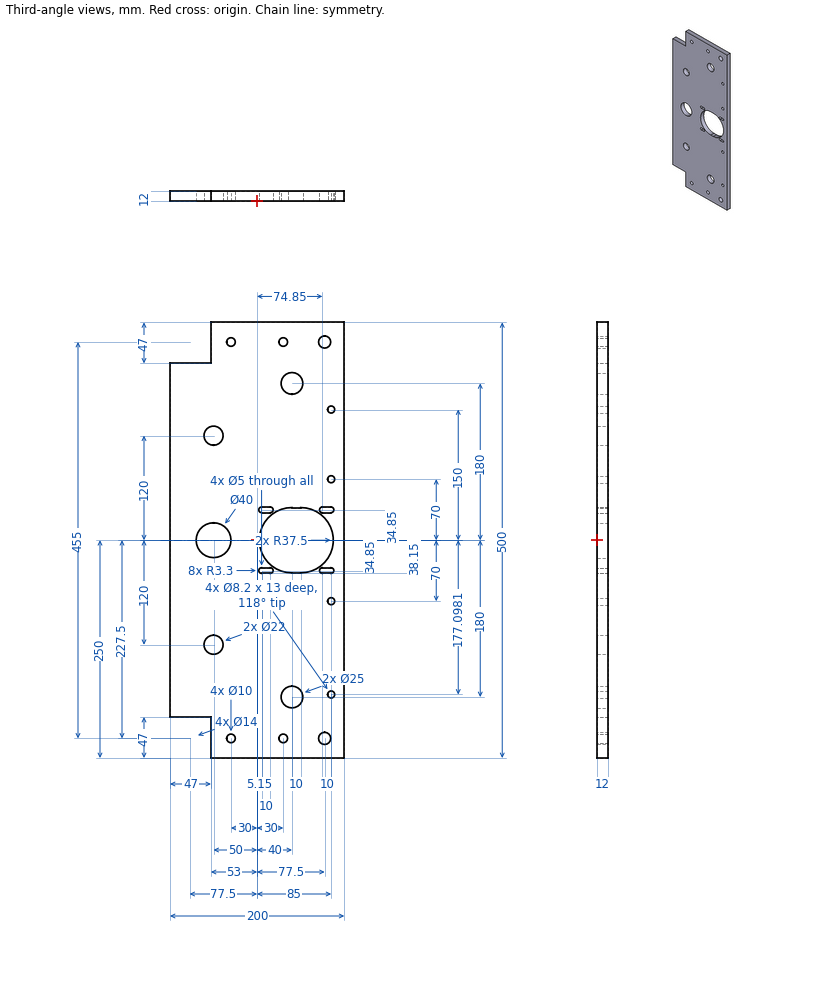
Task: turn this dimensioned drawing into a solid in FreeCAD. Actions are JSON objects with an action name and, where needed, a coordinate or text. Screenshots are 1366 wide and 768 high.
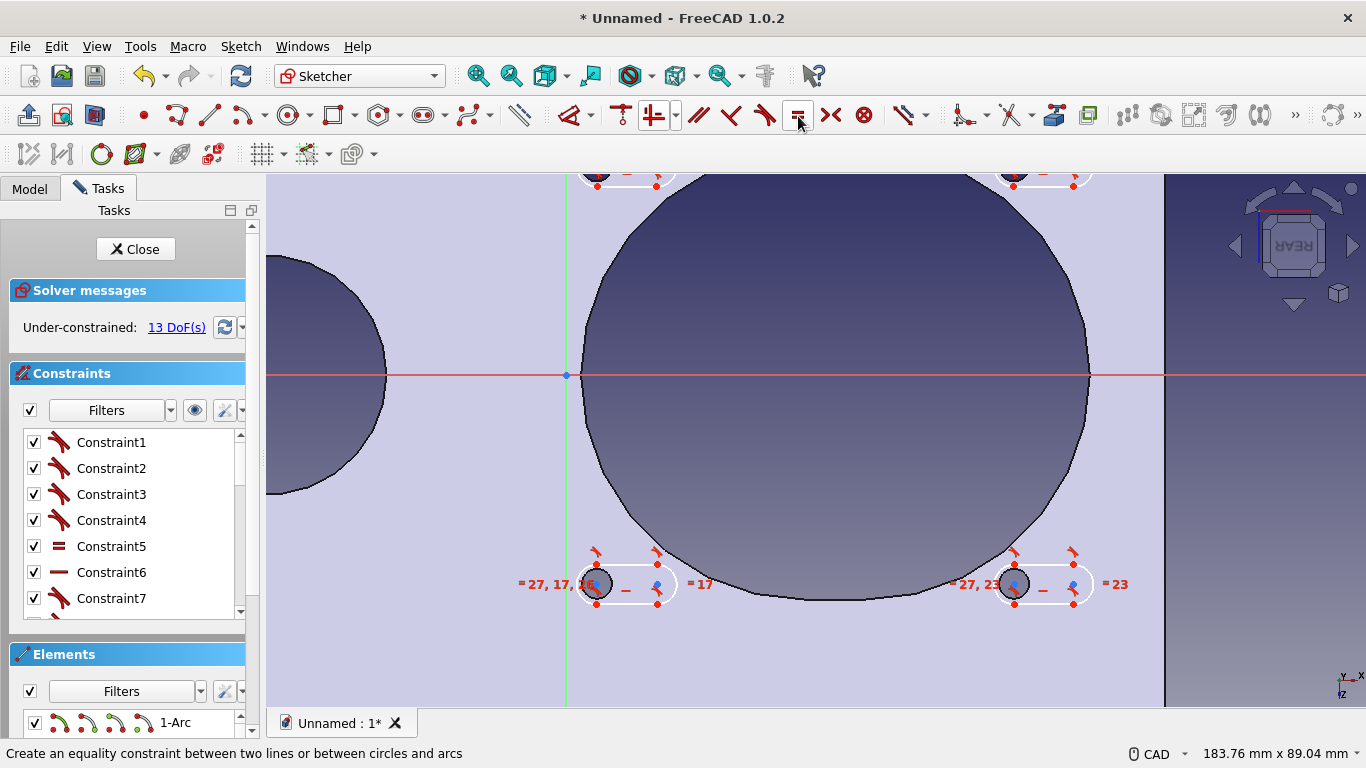
{"action": "scroll", "coordinate": [580, 573], "scroll_direction": "down", "scroll_amount": 2}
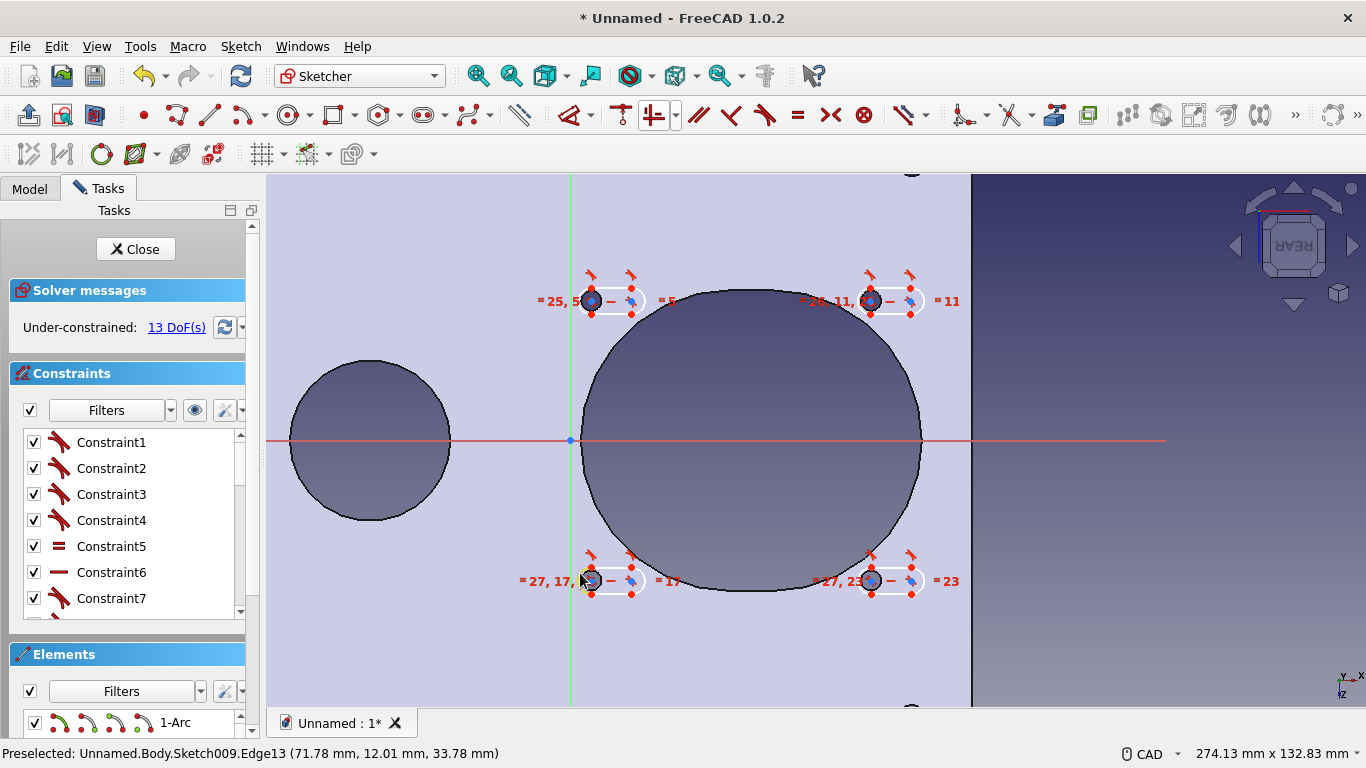
{"action": "left_click", "coordinate": [592, 301]}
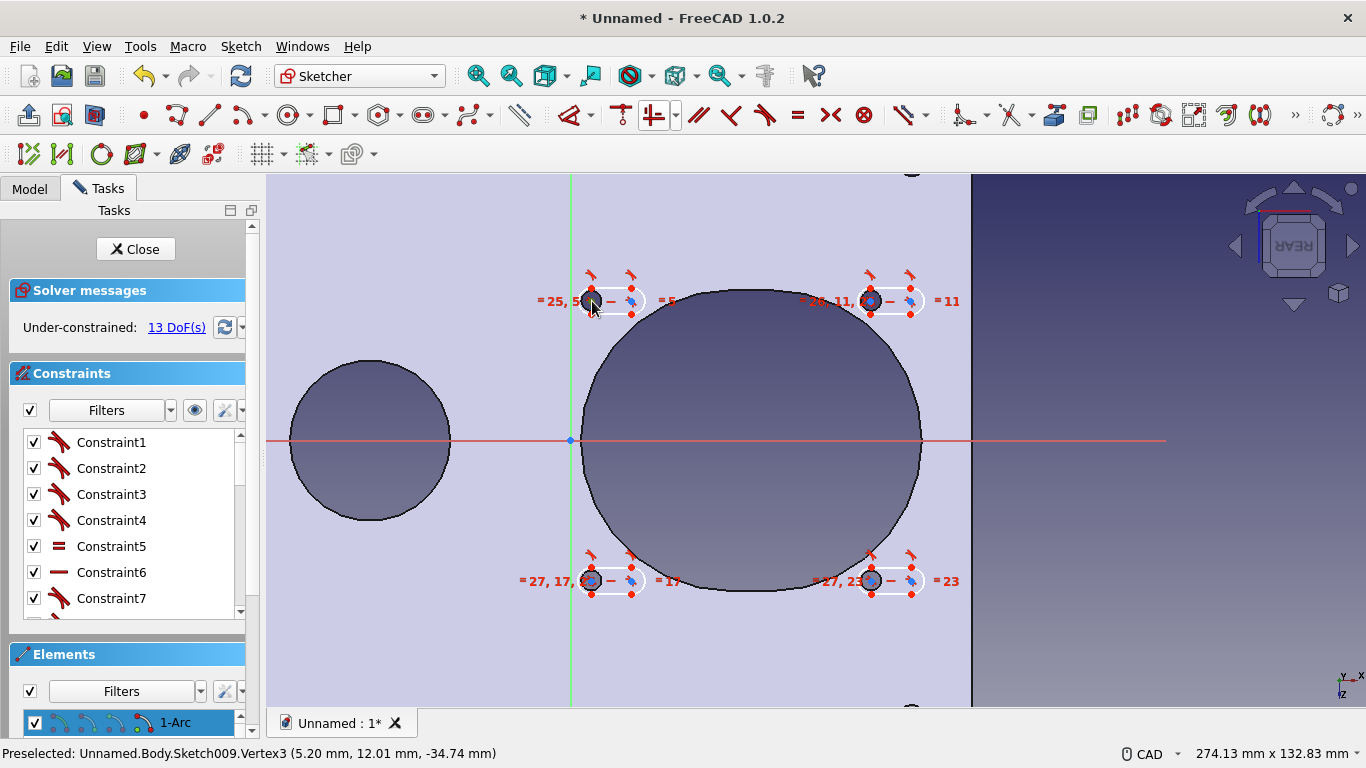
{"action": "left_click", "coordinate": [591, 581]}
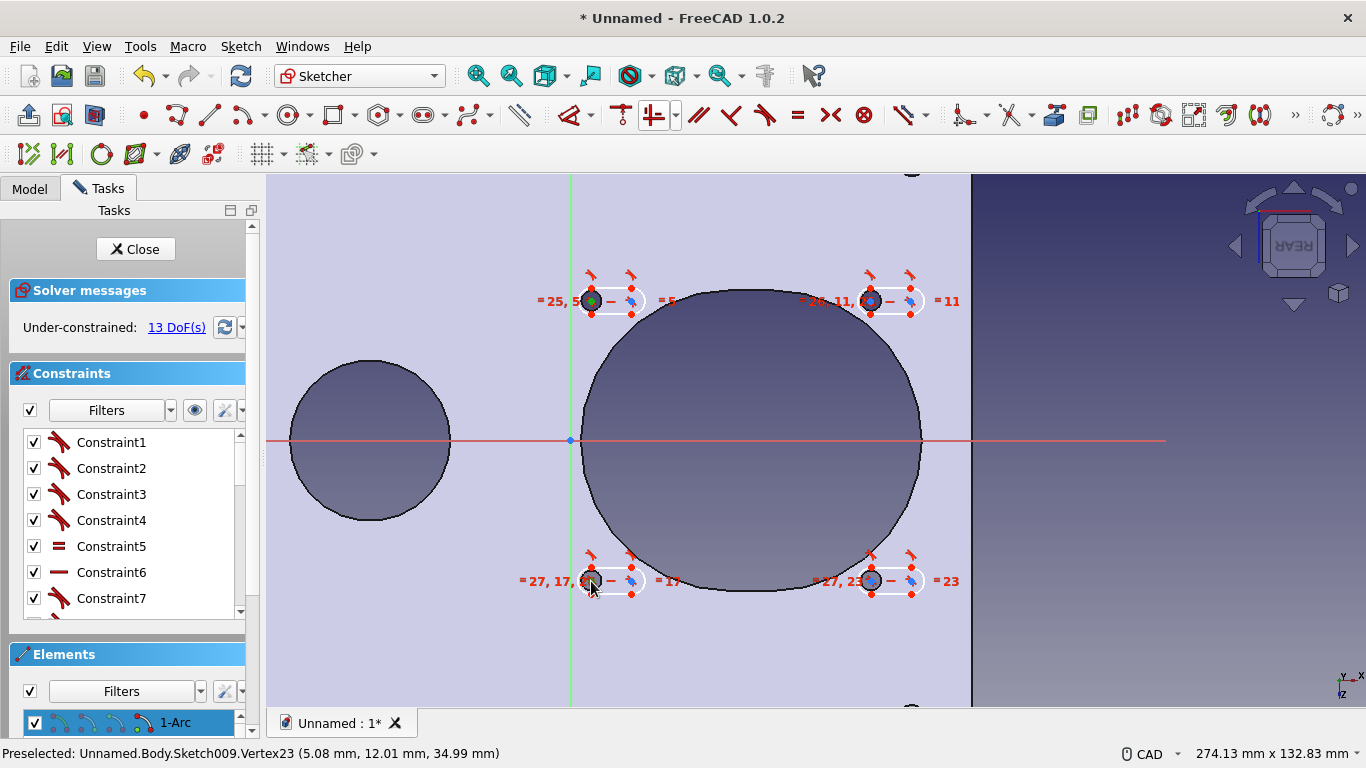
{"action": "left_click", "coordinate": [359, 441]}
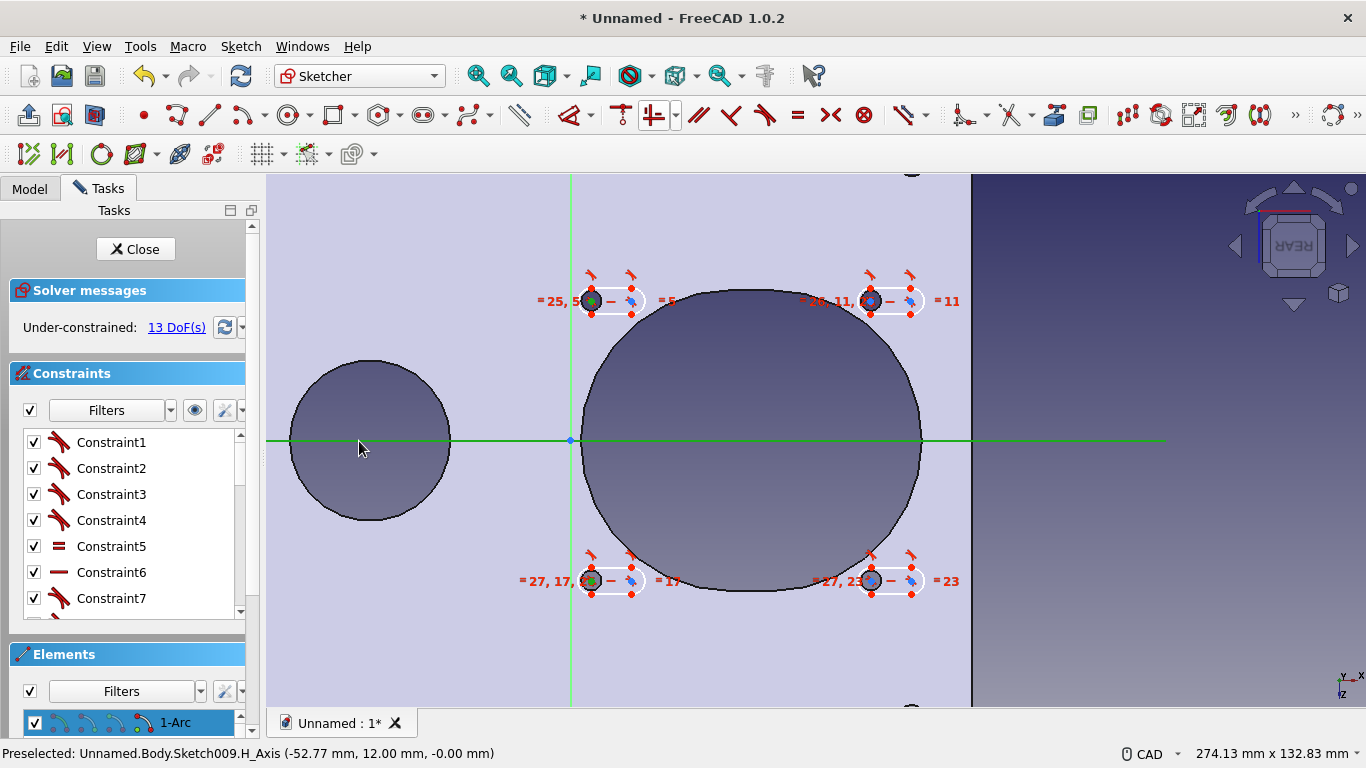
{"action": "key", "text": "s"}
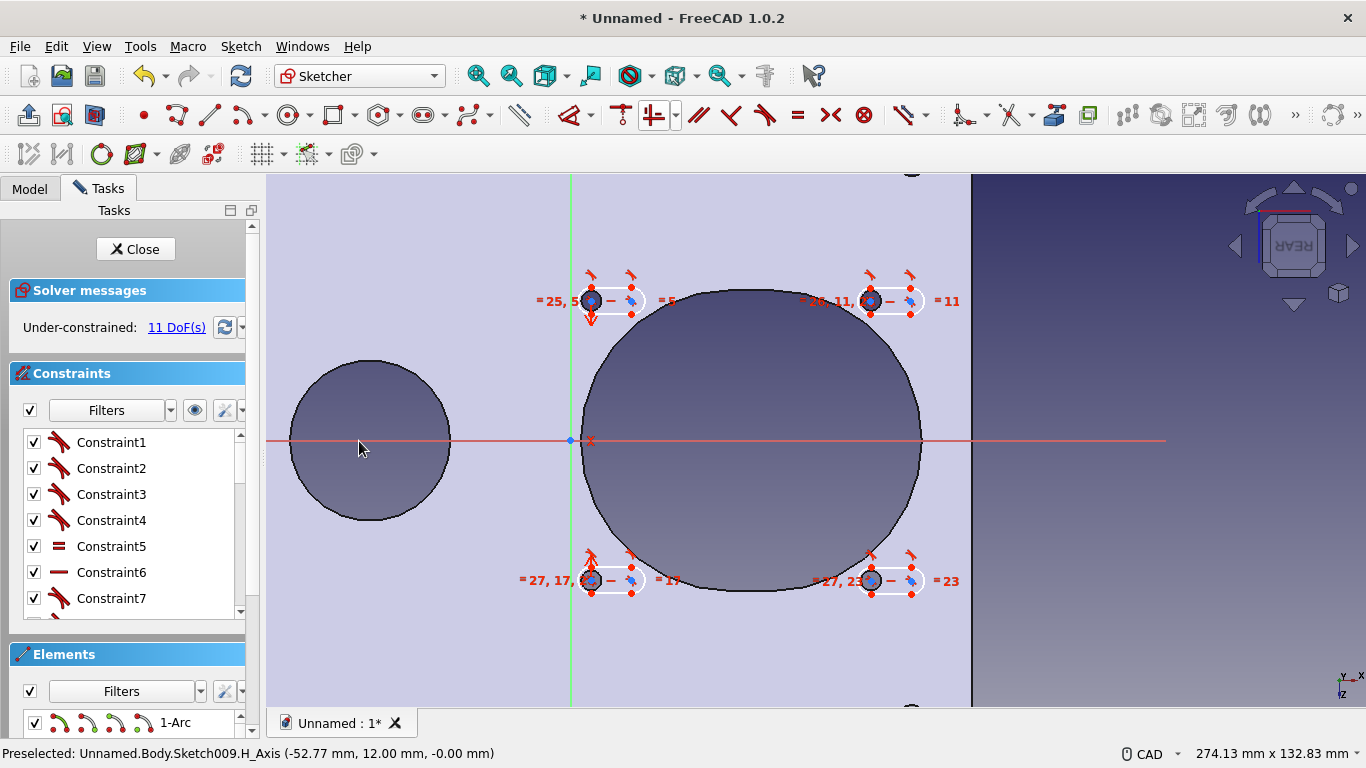
{"action": "left_click", "coordinate": [871, 301]}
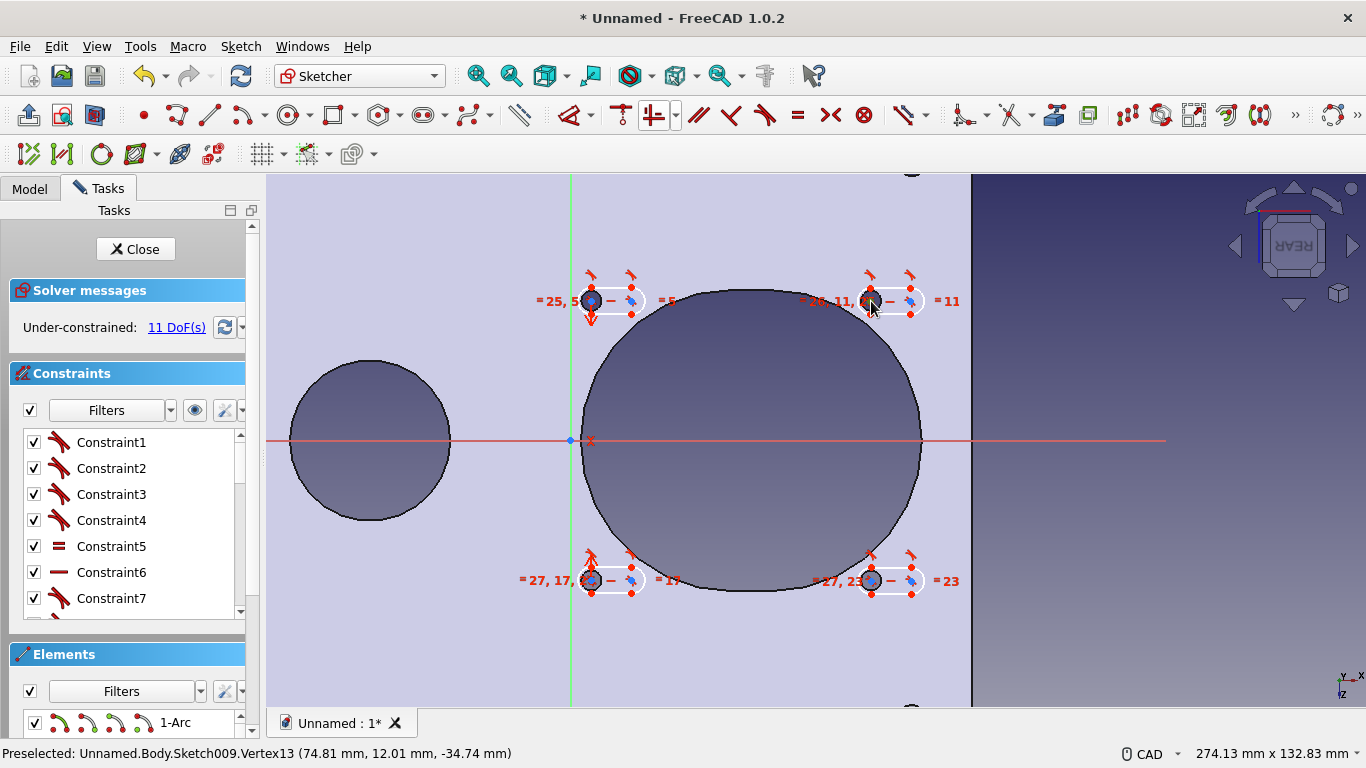
{"action": "left_click", "coordinate": [871, 581]}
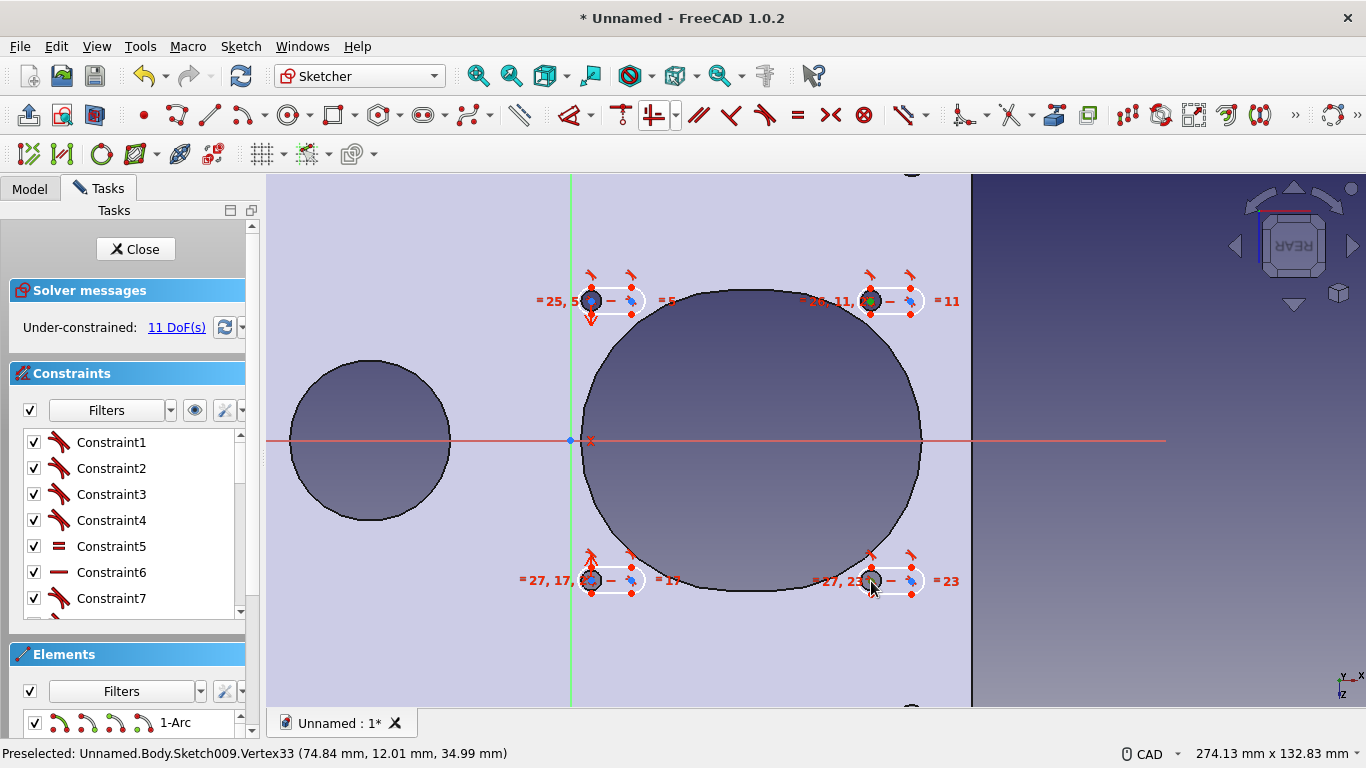
{"action": "left_click", "coordinate": [359, 441]}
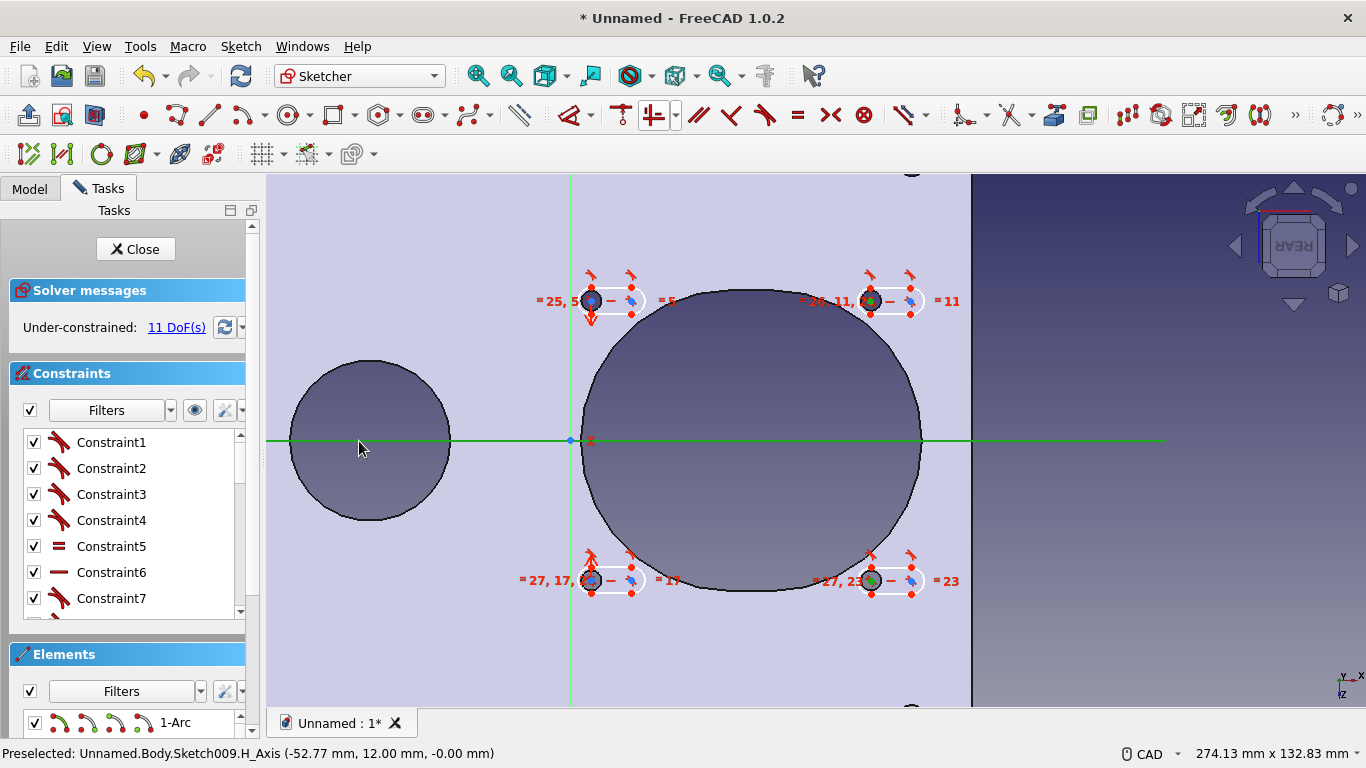
{"action": "key", "text": "s"}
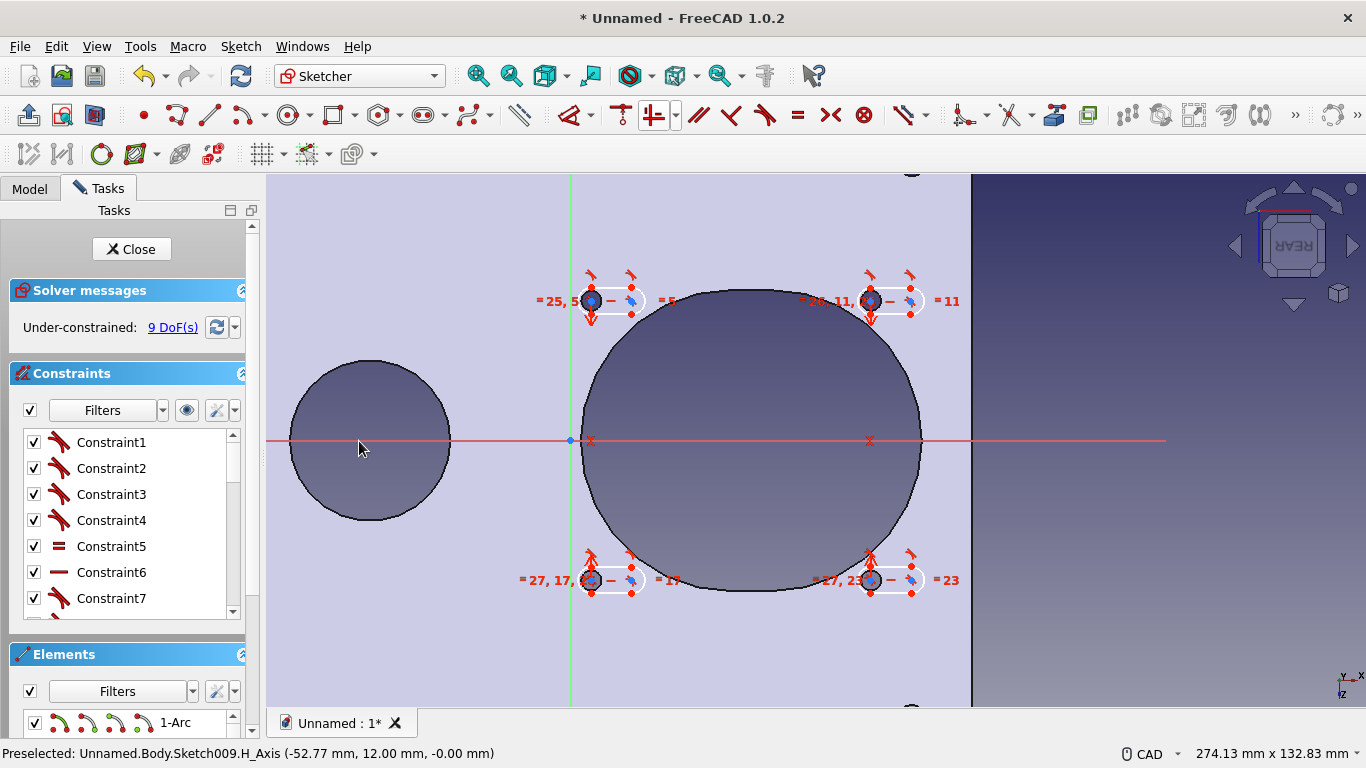
{"action": "key", "text": "d"}